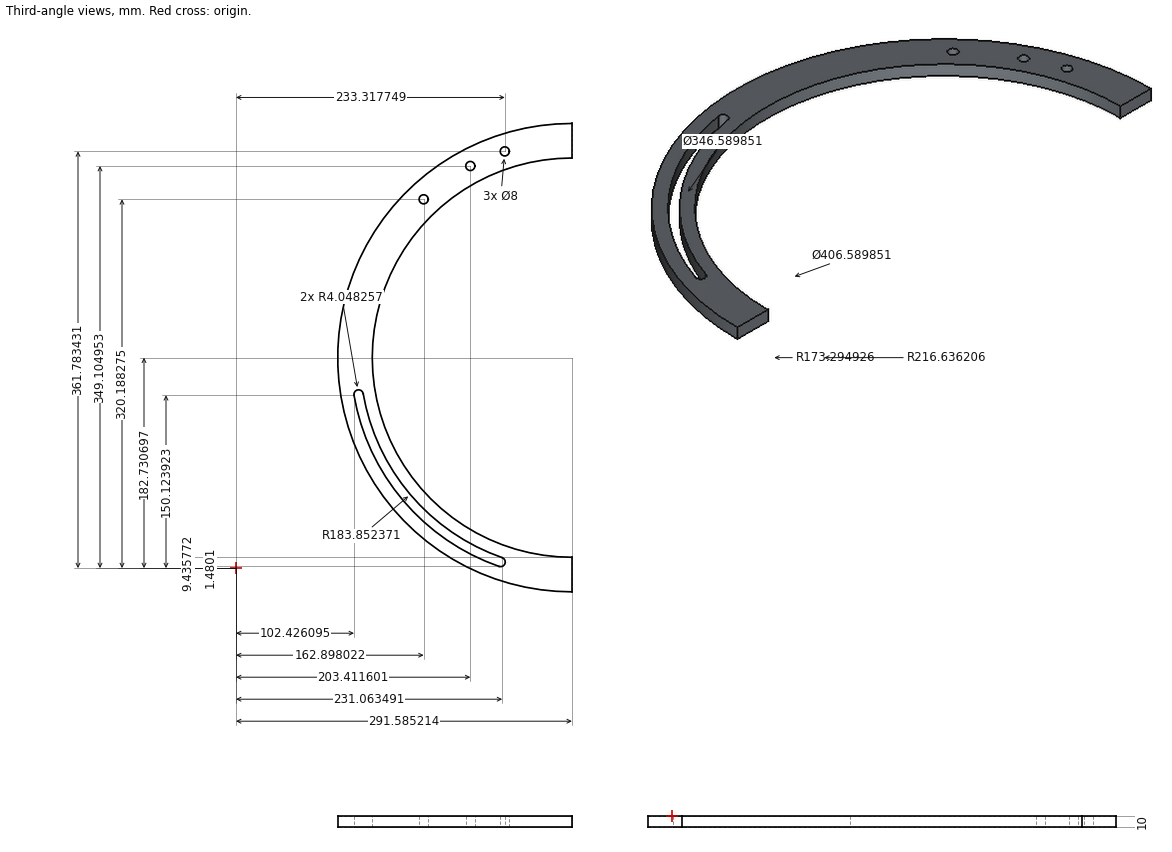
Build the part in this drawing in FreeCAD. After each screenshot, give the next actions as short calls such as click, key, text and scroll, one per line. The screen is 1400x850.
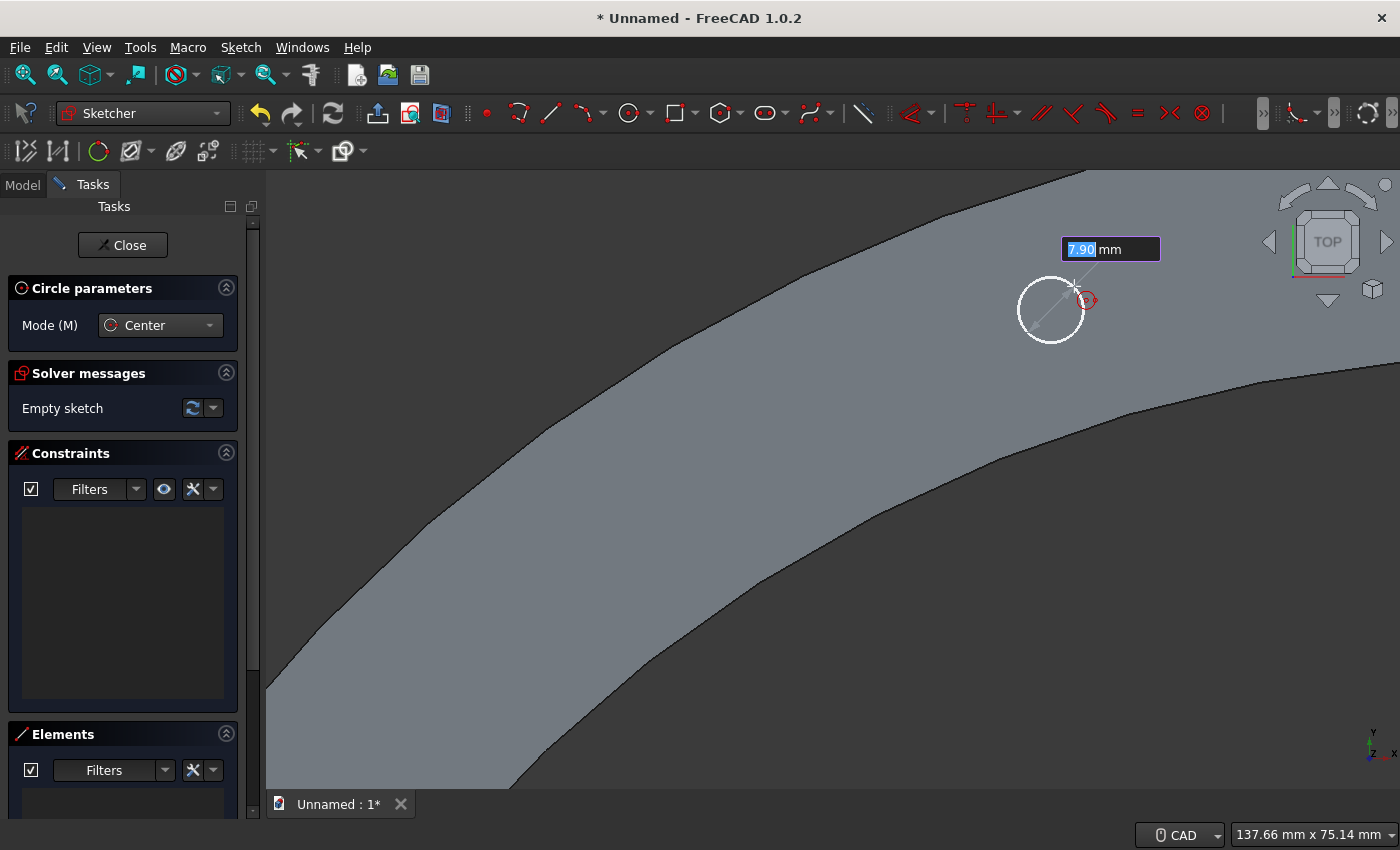
text(8)
key(Return)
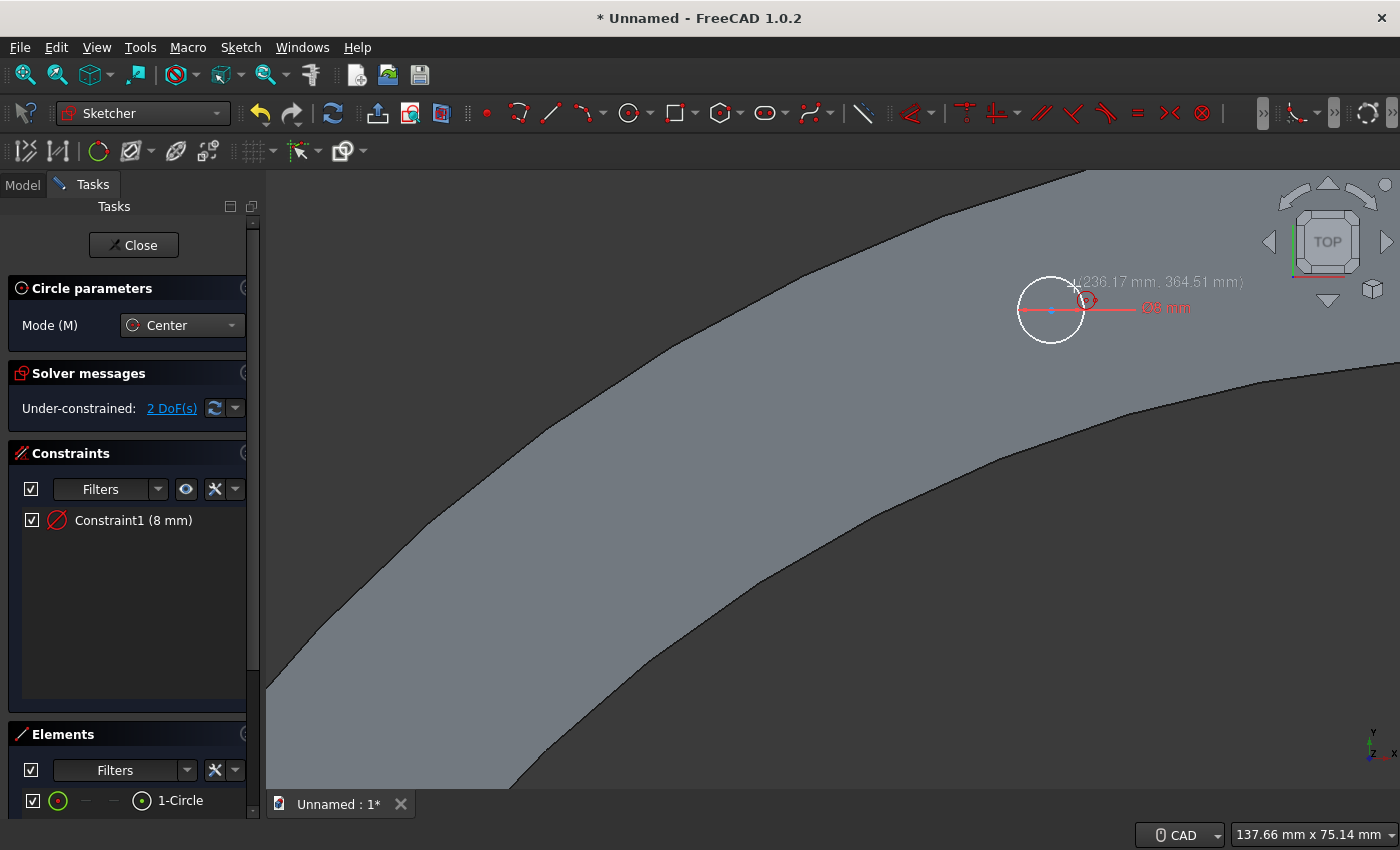
click(804, 414)
move(827, 391)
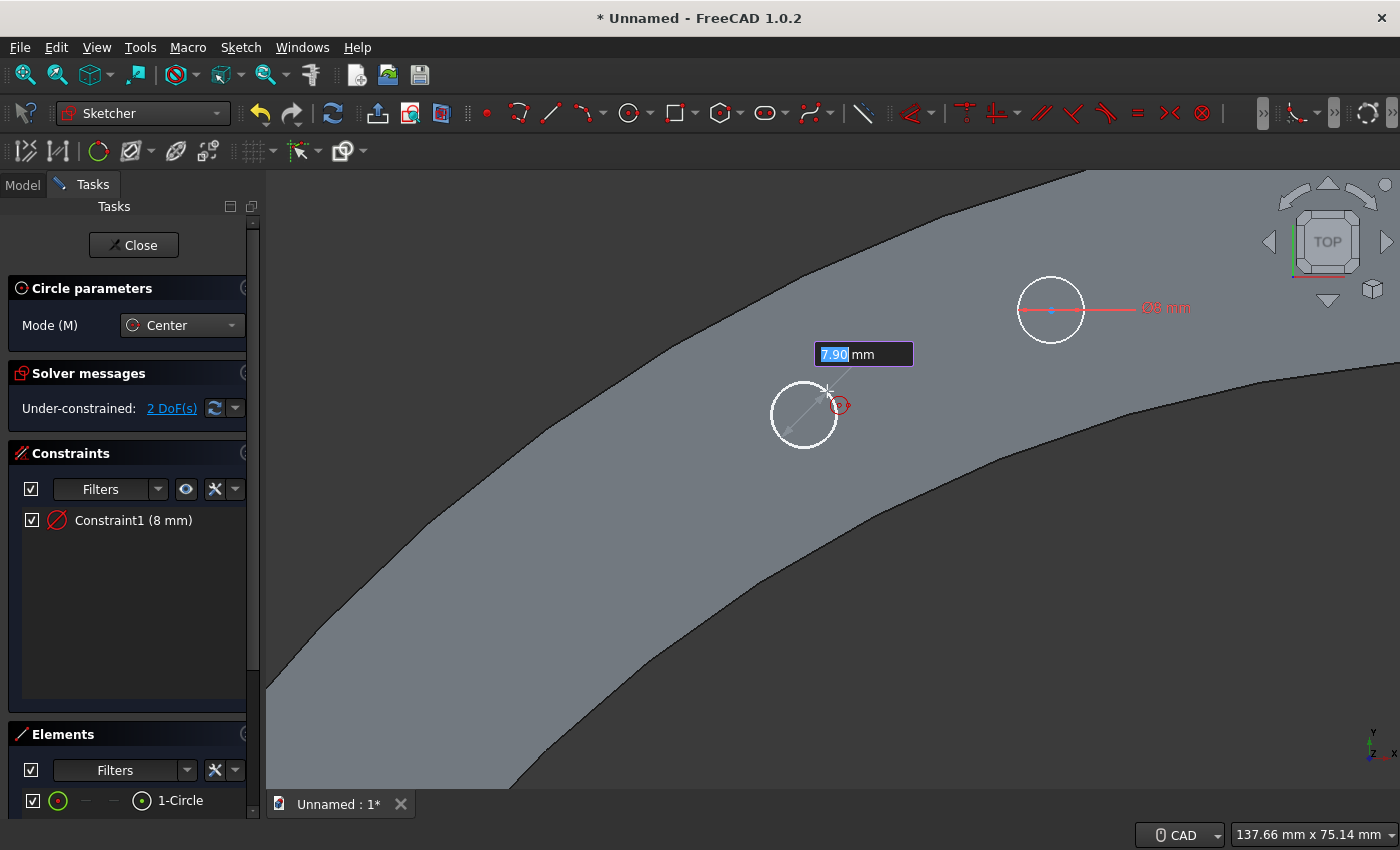
text(8)
key(Return)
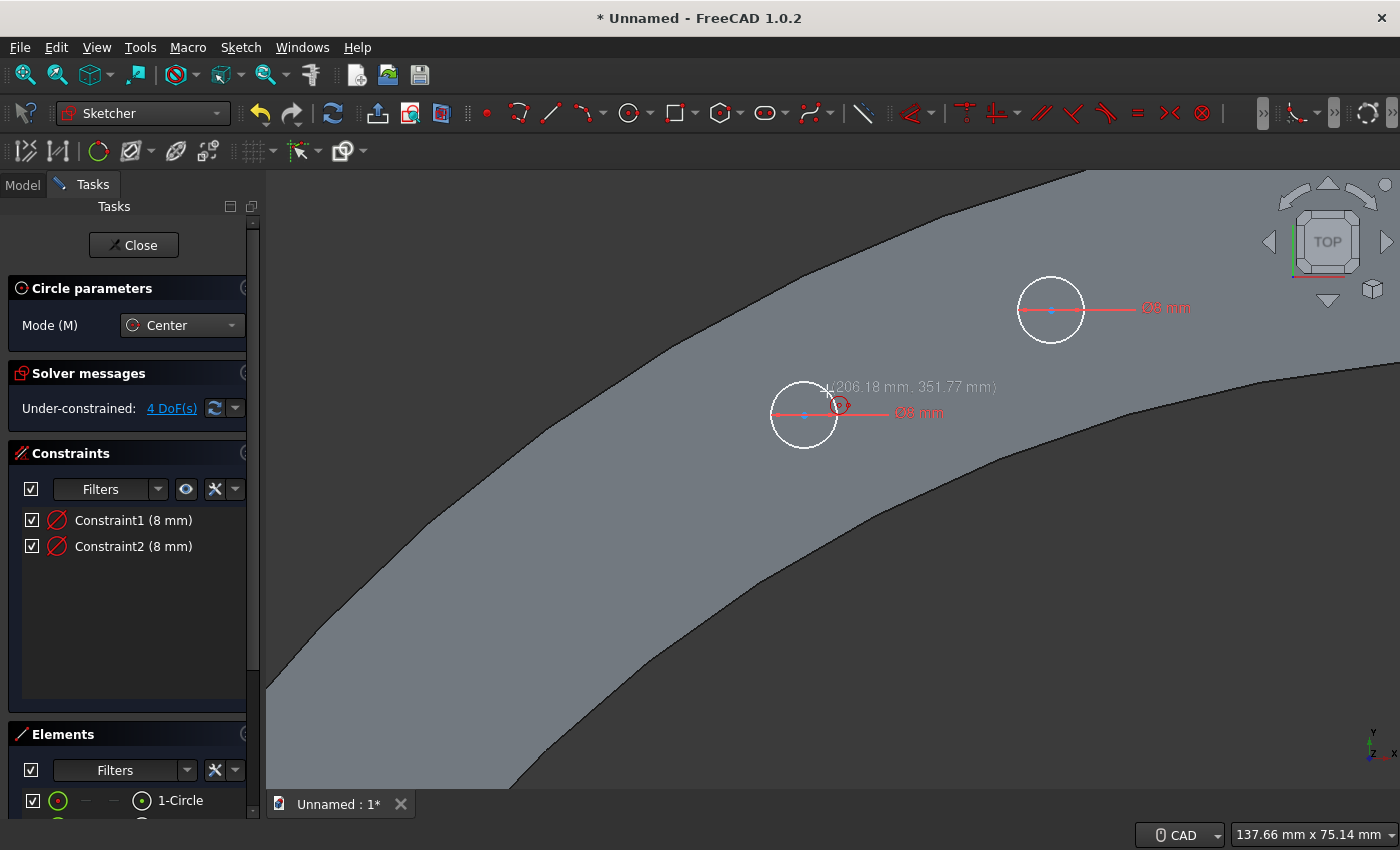
click(470, 652)
move(494, 629)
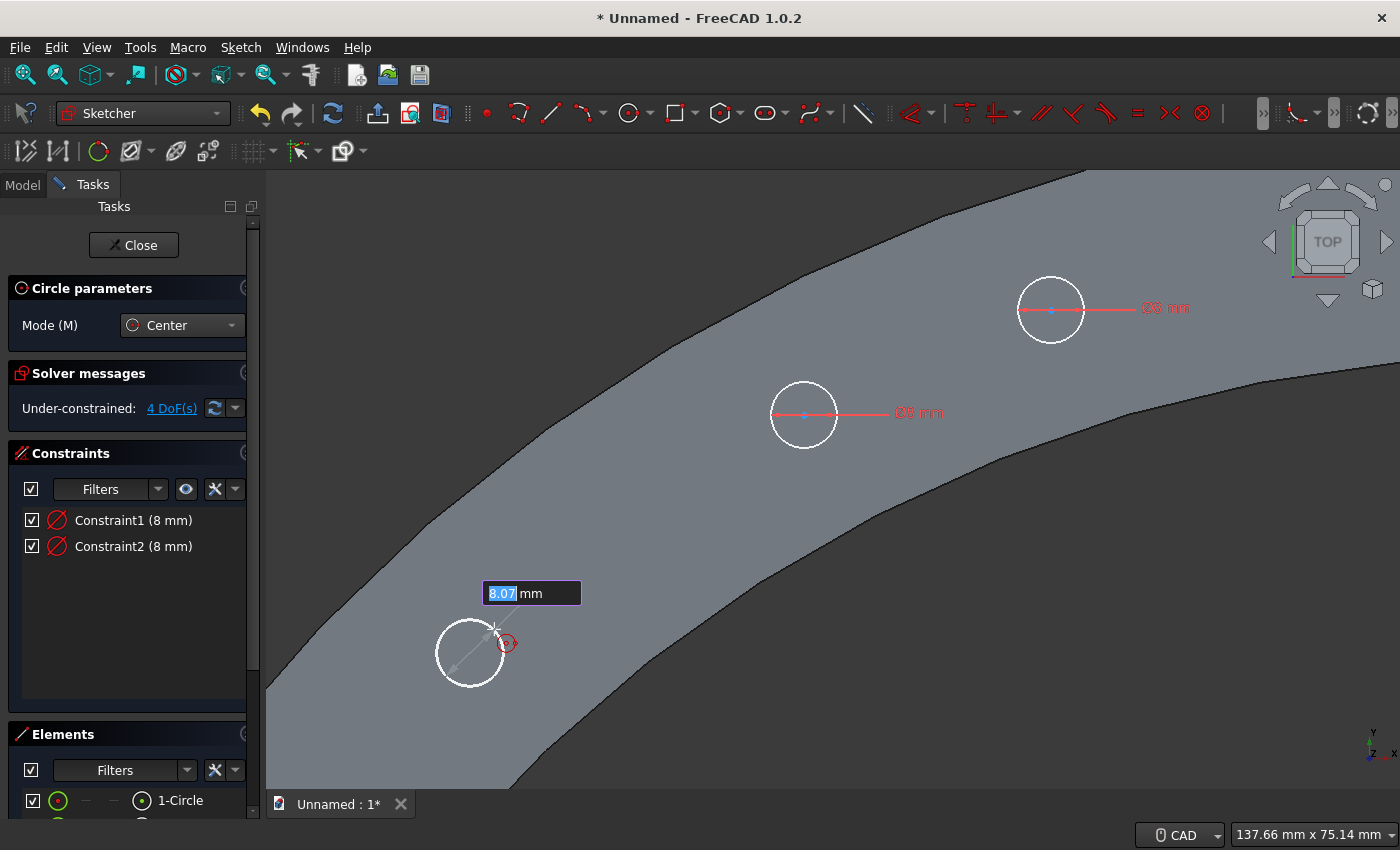
text(8)
key(Return)
key(Escape)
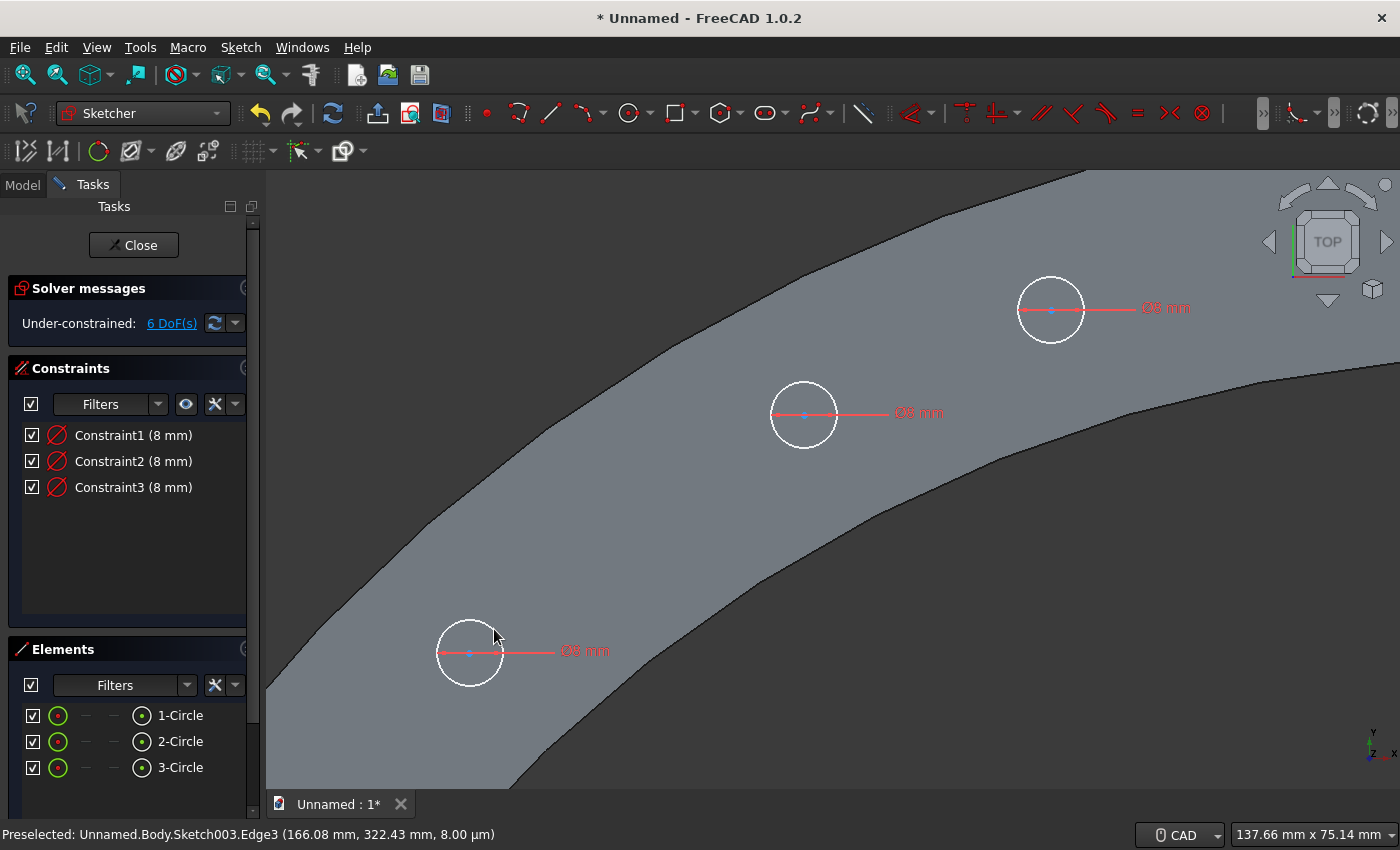
click(910, 114)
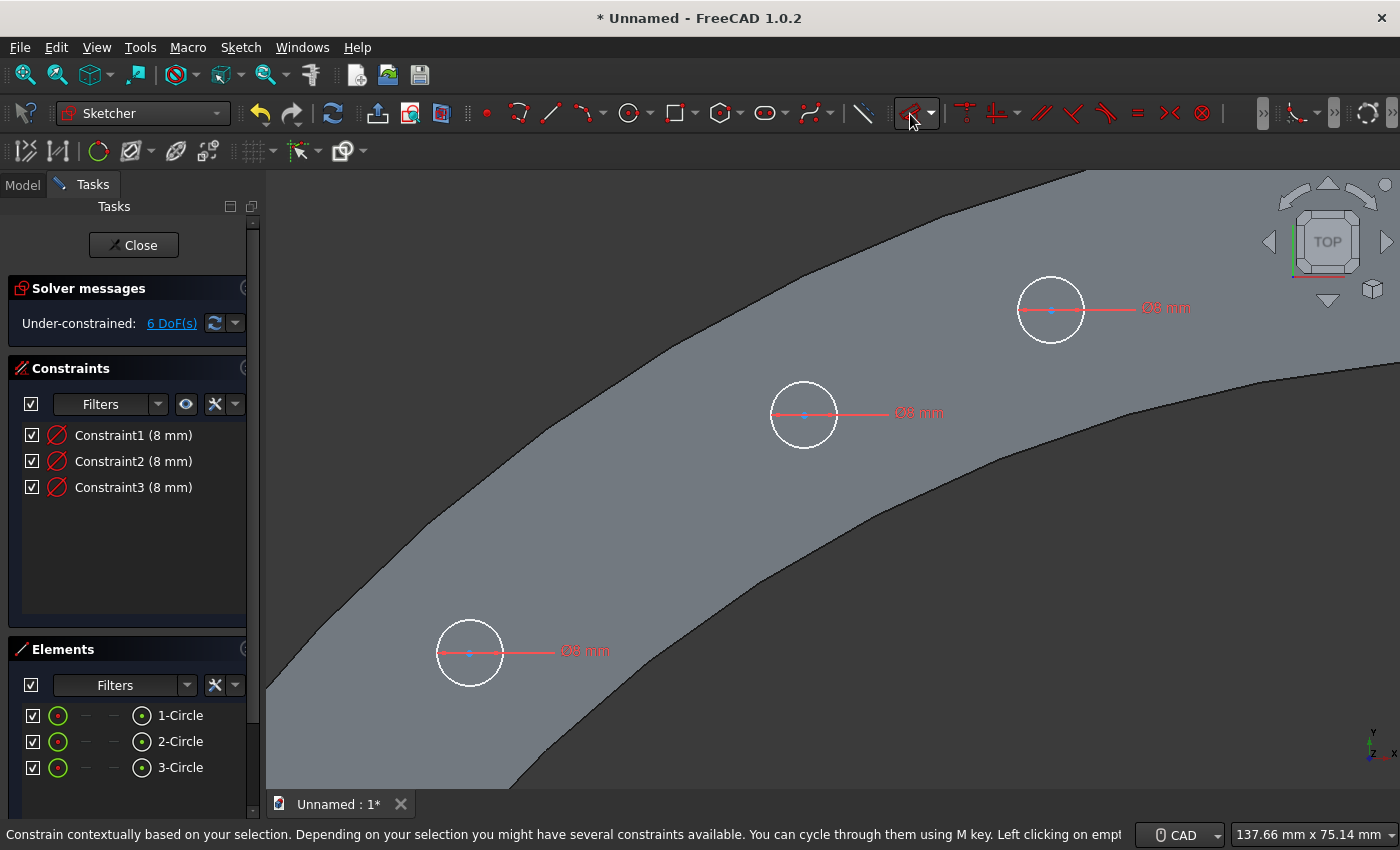
click(1051, 310)
click(672, 276)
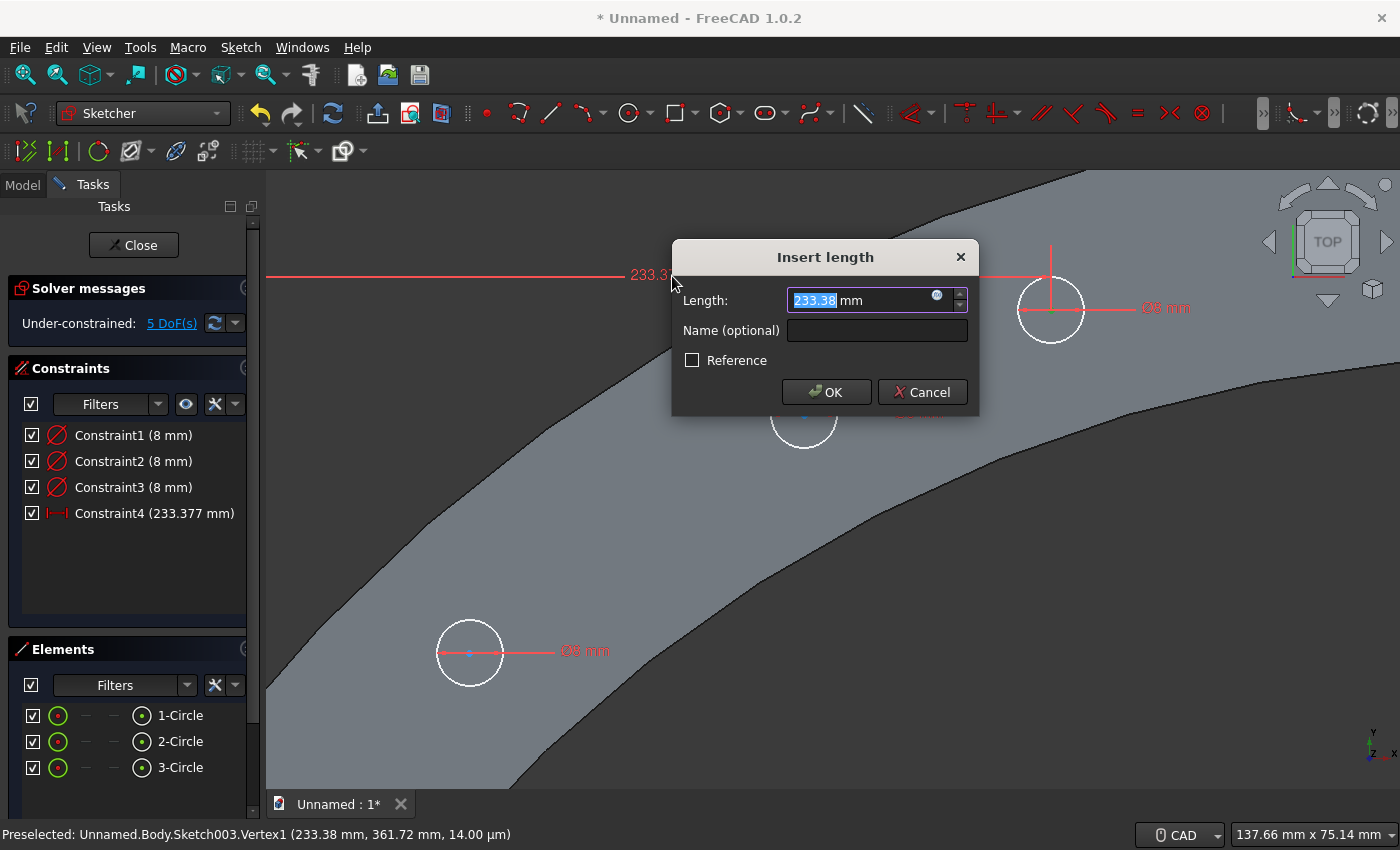
text(233.317749)
key(Return)